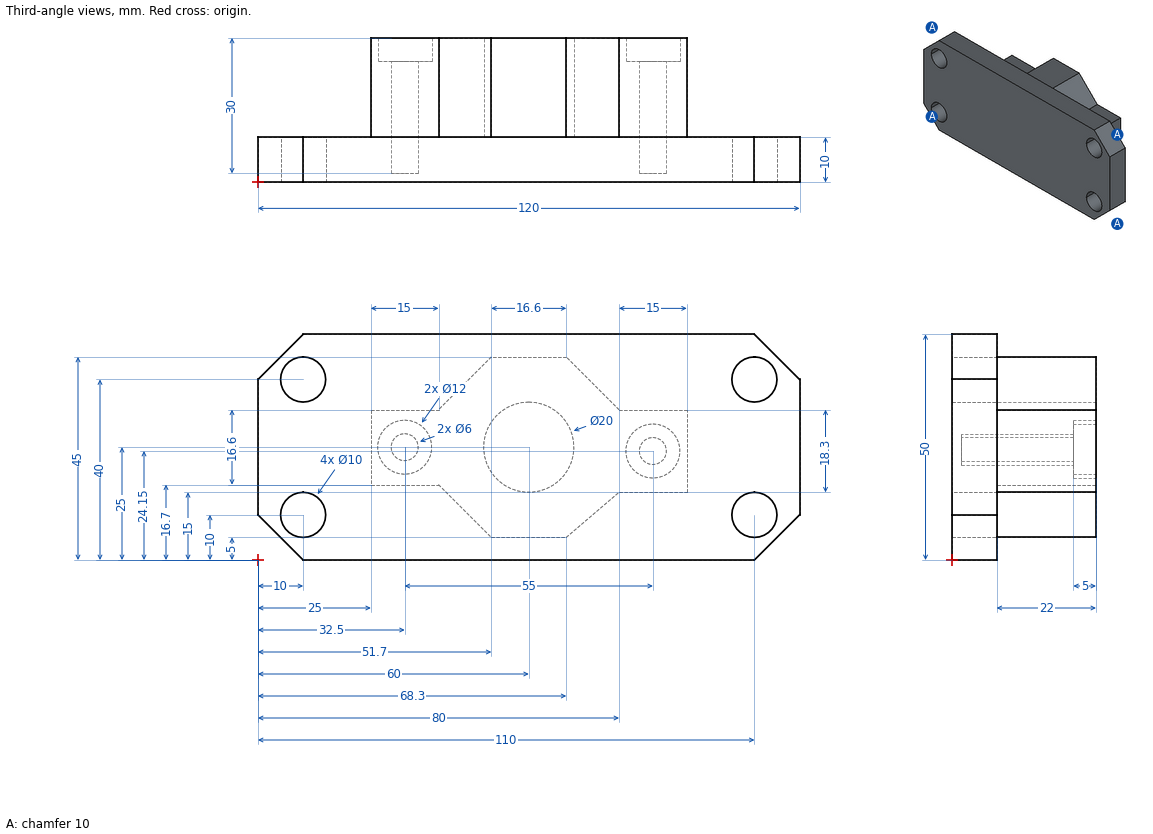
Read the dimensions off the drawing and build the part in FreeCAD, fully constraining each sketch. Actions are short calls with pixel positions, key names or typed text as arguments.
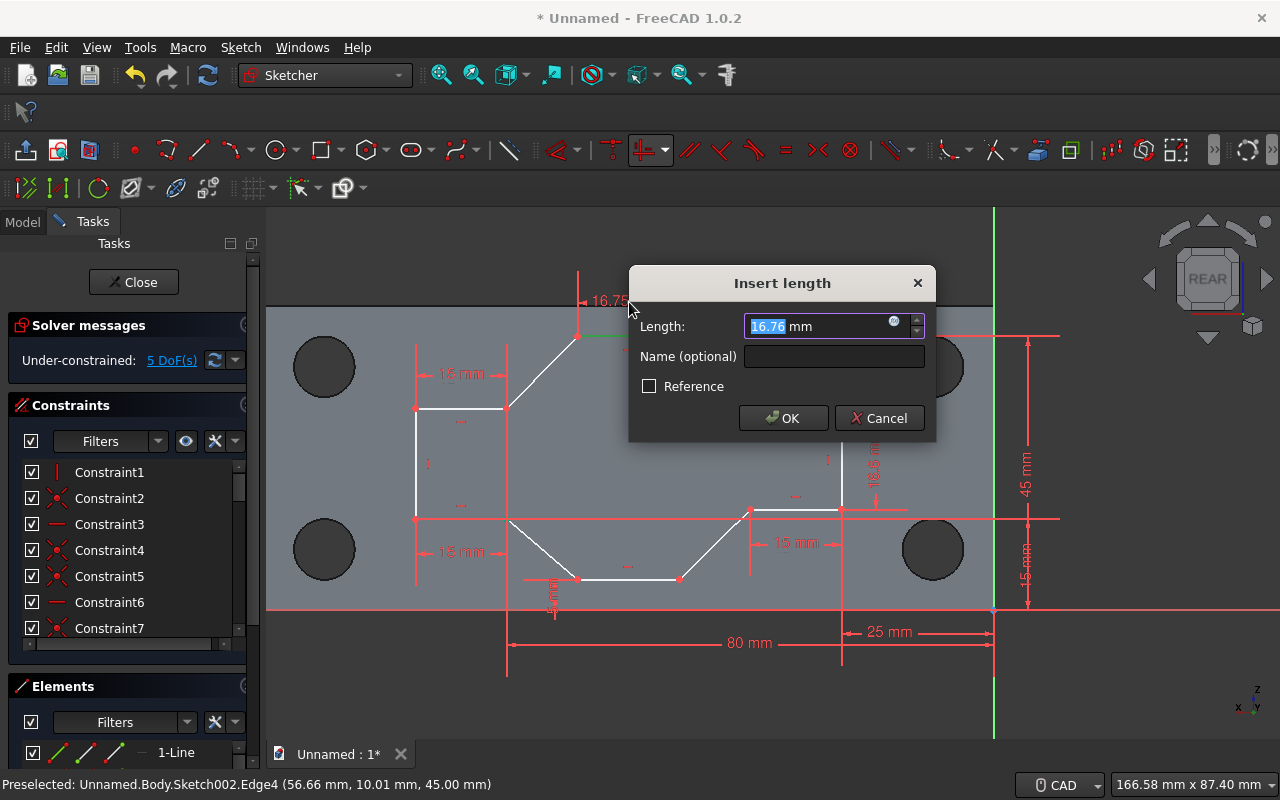
text(16.6)
key(Return)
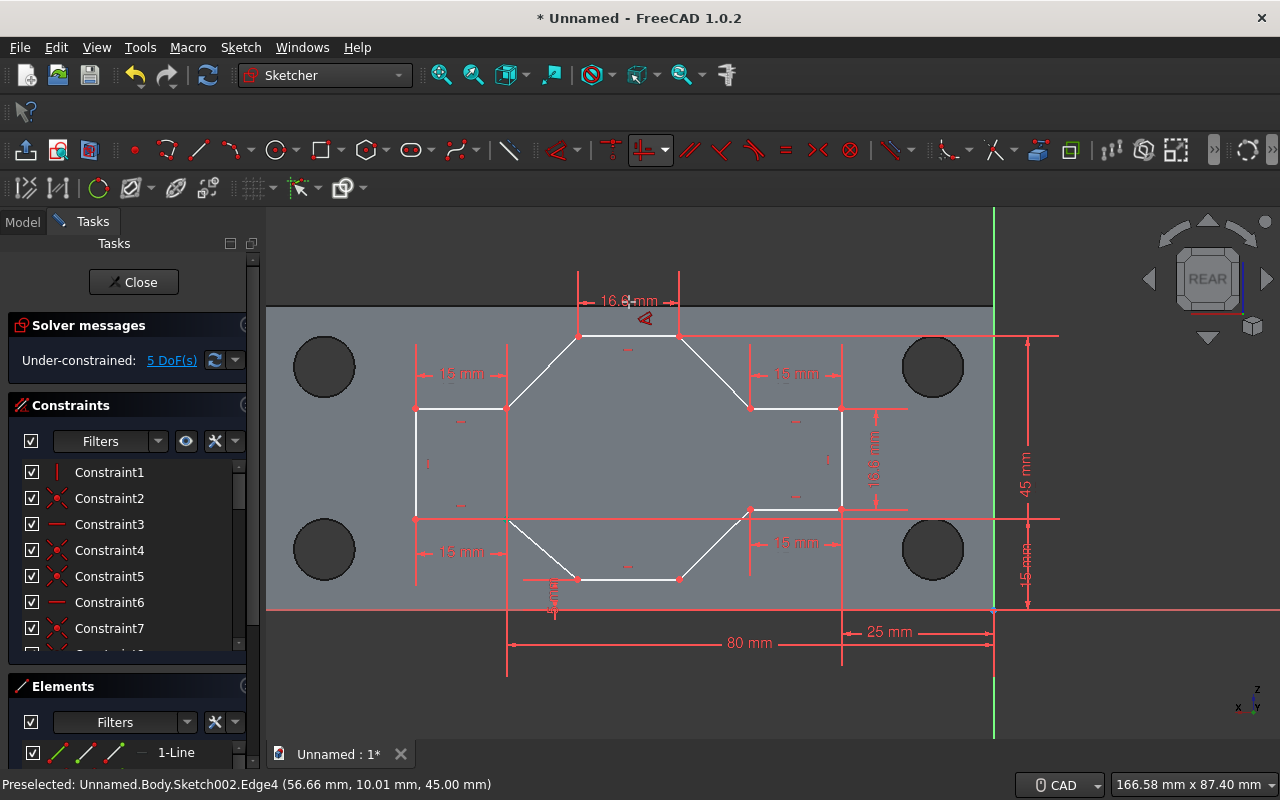
click(416, 442)
click(382, 464)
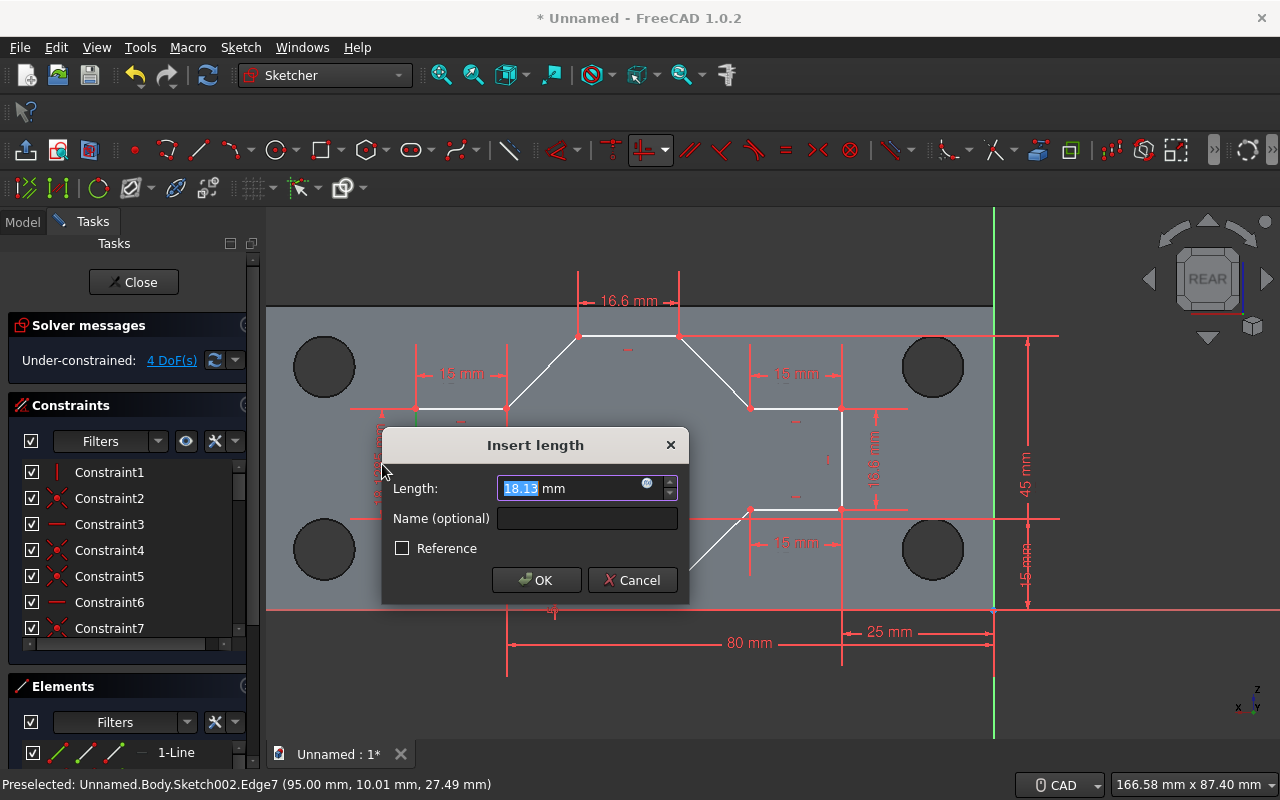
text(18.3)
key(Return)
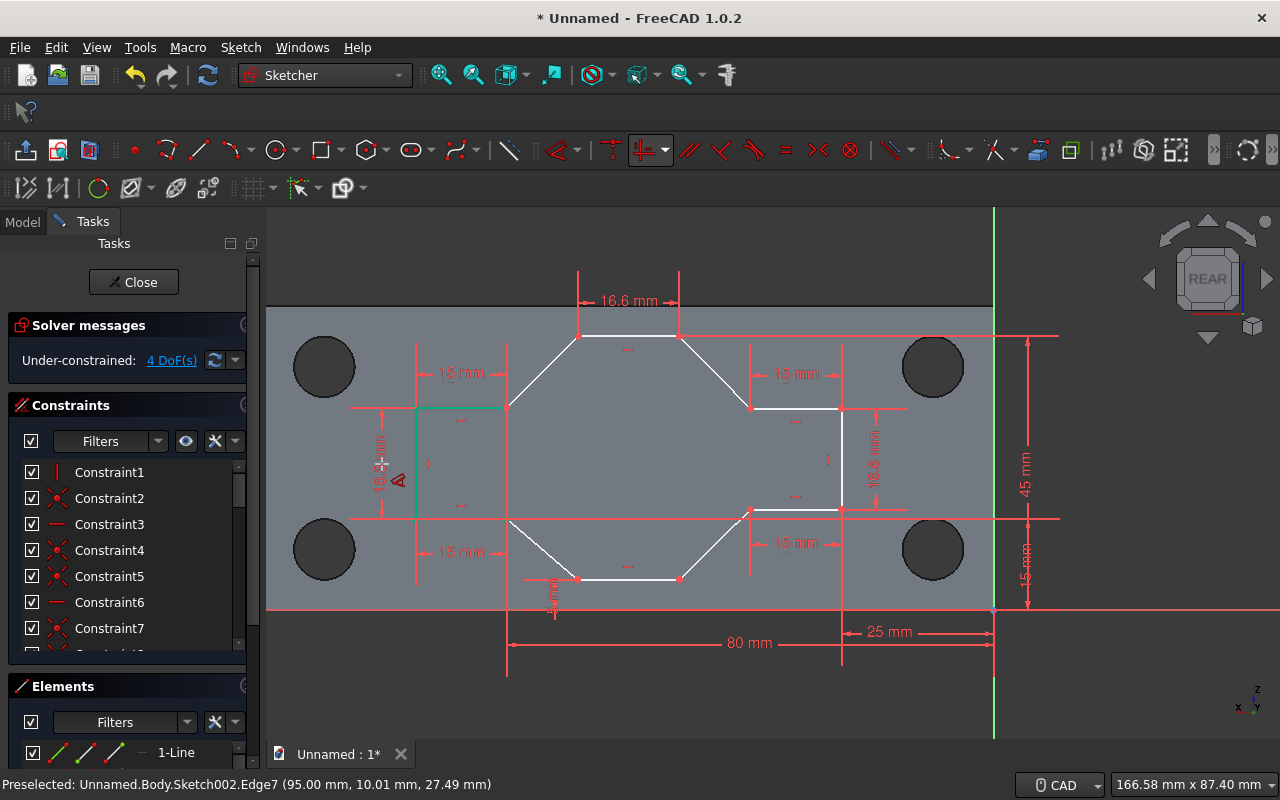
click(608, 580)
click(629, 546)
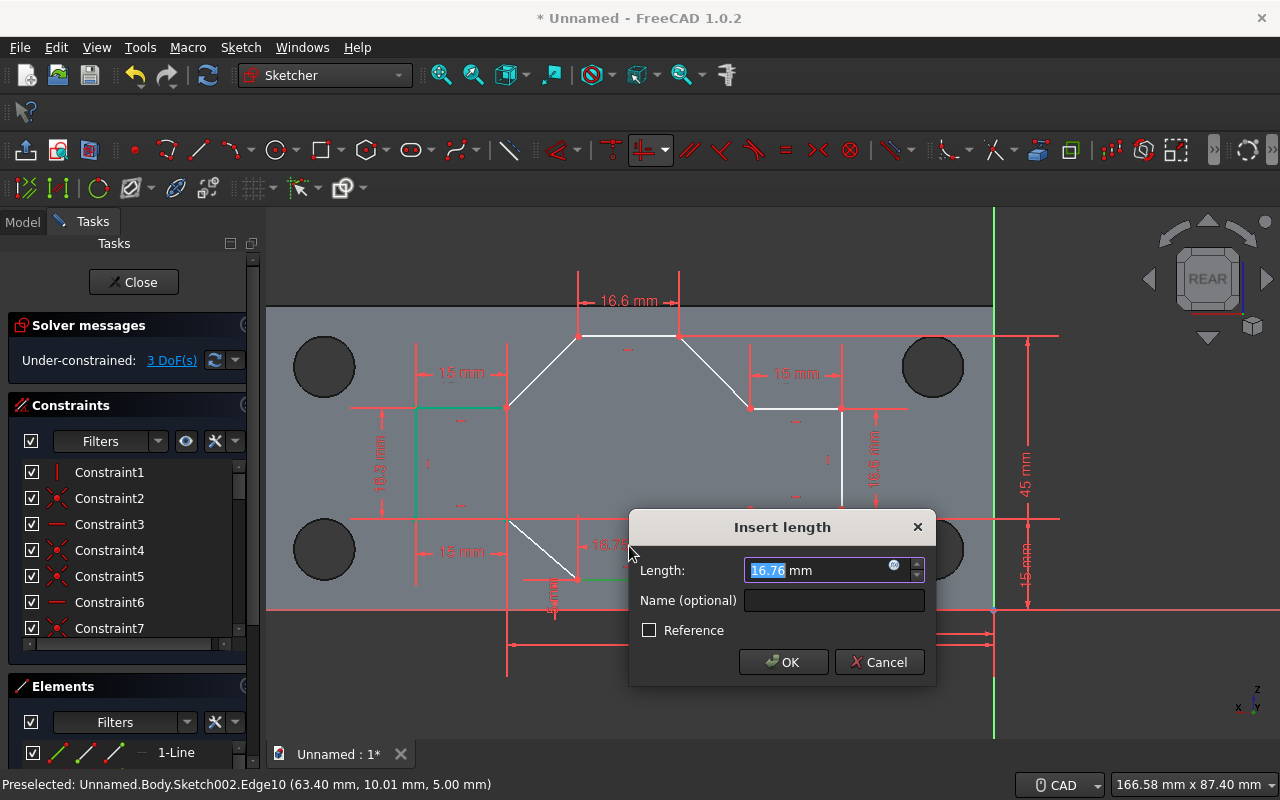
text(16.6)
key(Return)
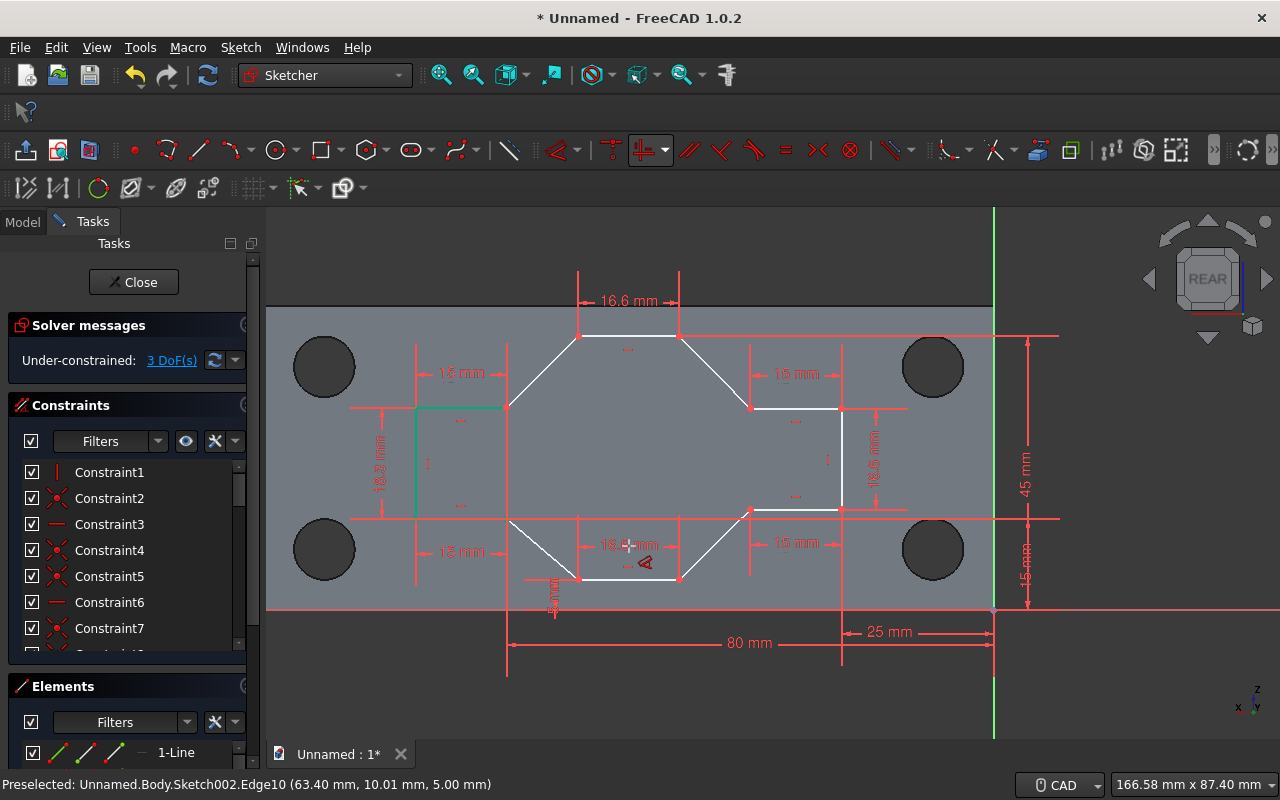
click(842, 510)
click(1028, 537)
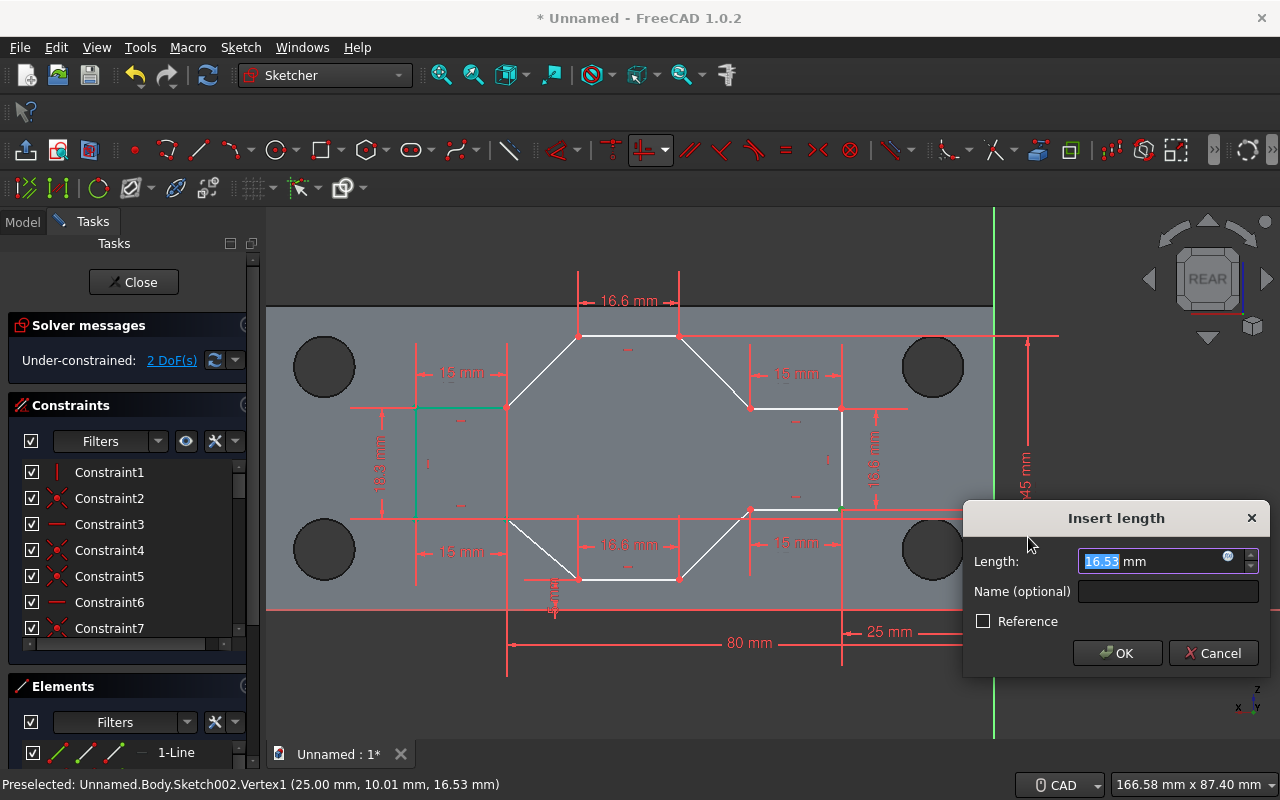
text(16.7)
key(Return)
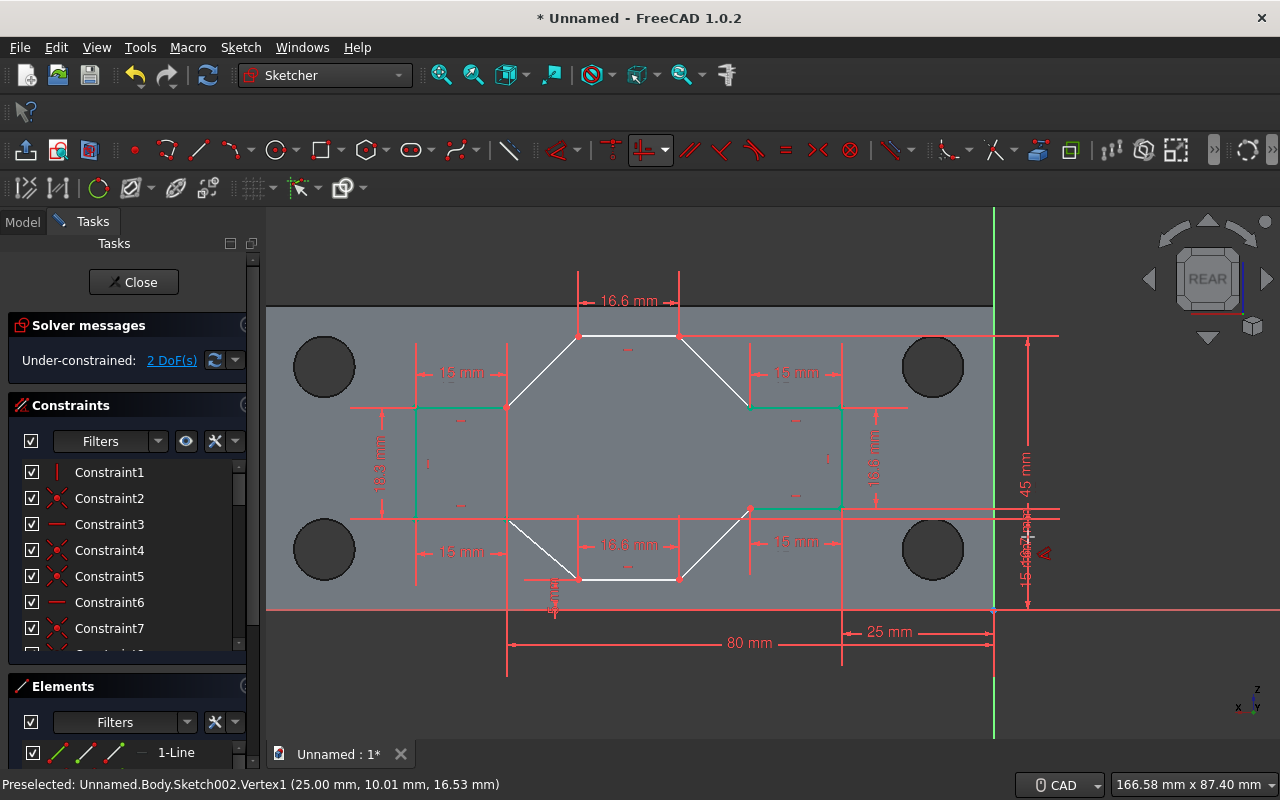
click(679, 336)
click(837, 302)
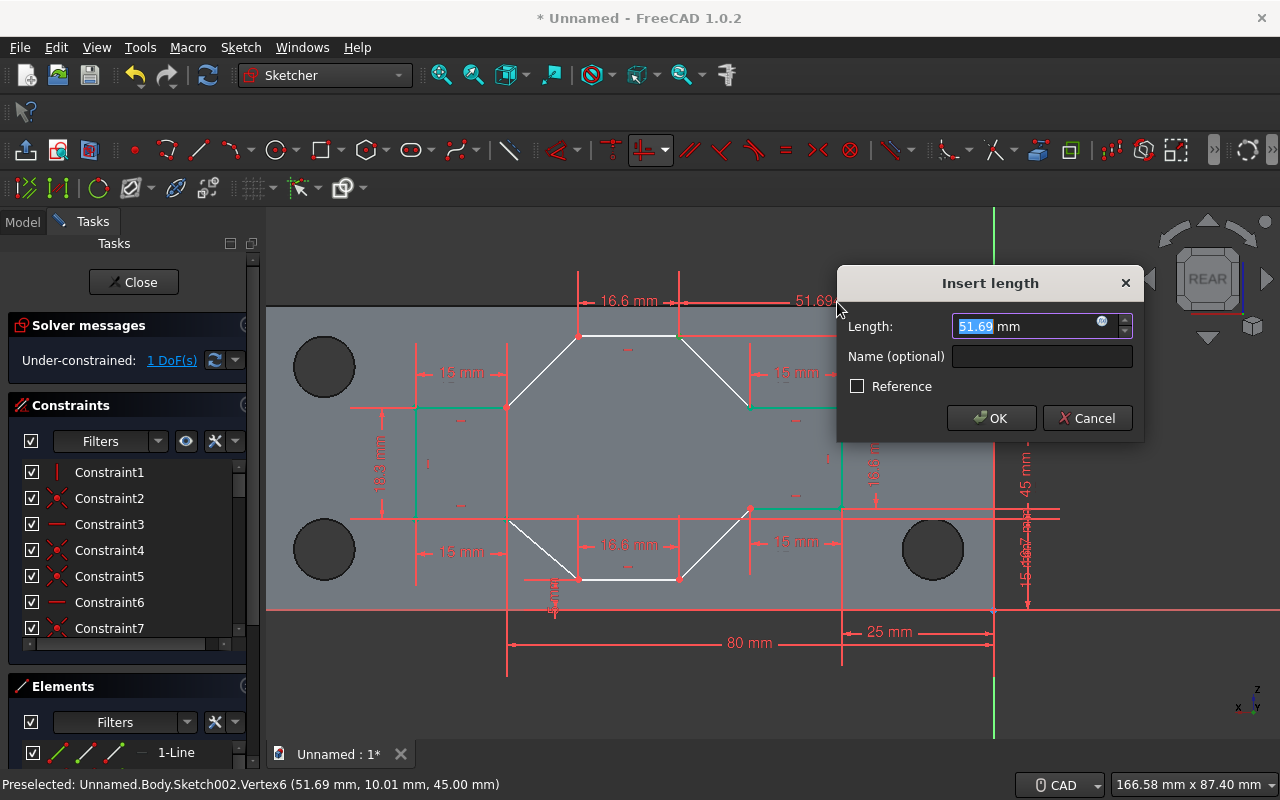
text(51.7)
key(Return)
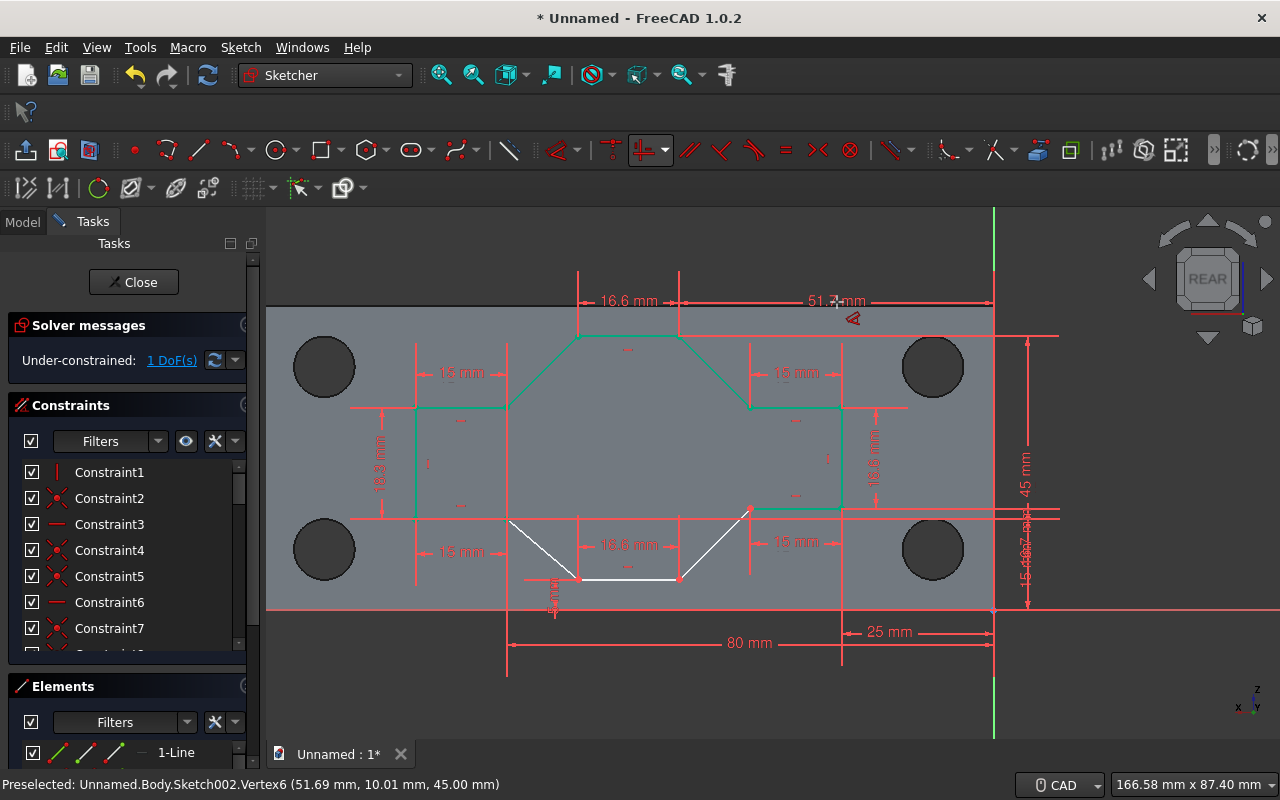
click(578, 580)
click(641, 644)